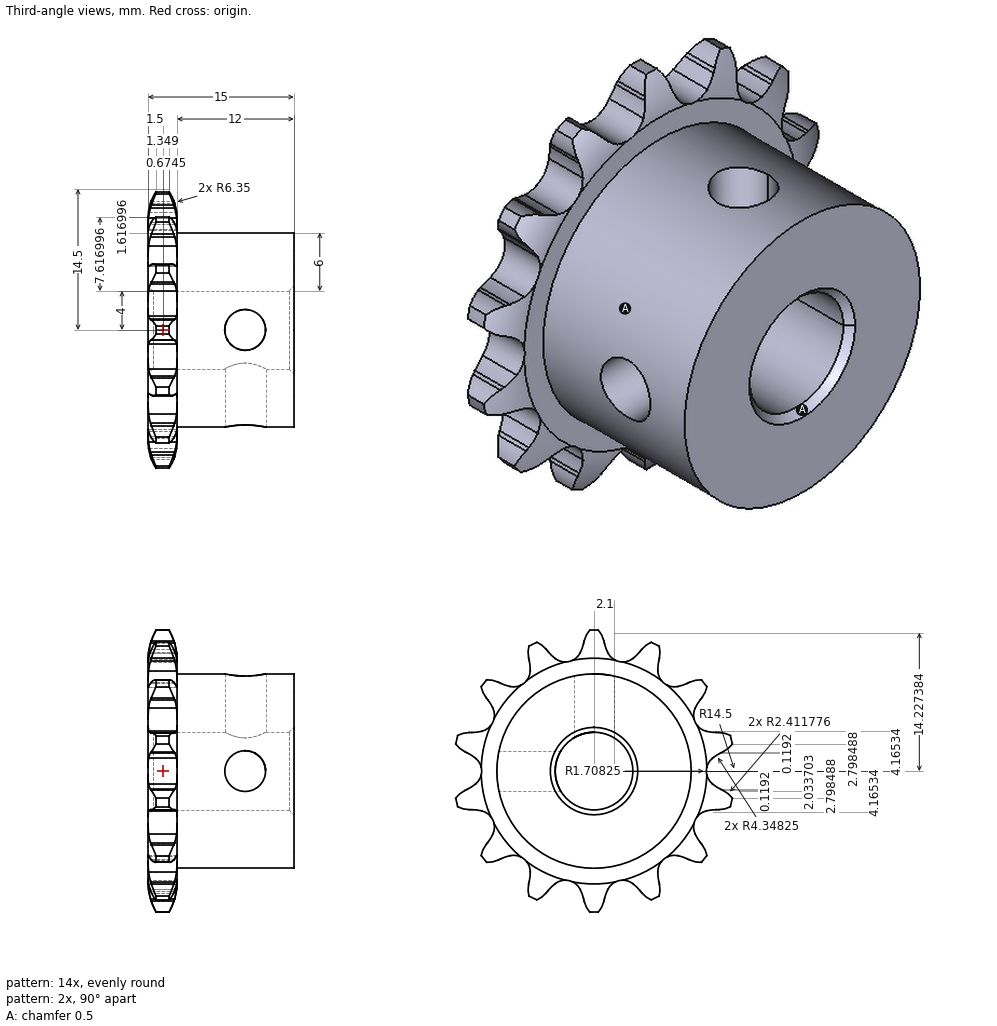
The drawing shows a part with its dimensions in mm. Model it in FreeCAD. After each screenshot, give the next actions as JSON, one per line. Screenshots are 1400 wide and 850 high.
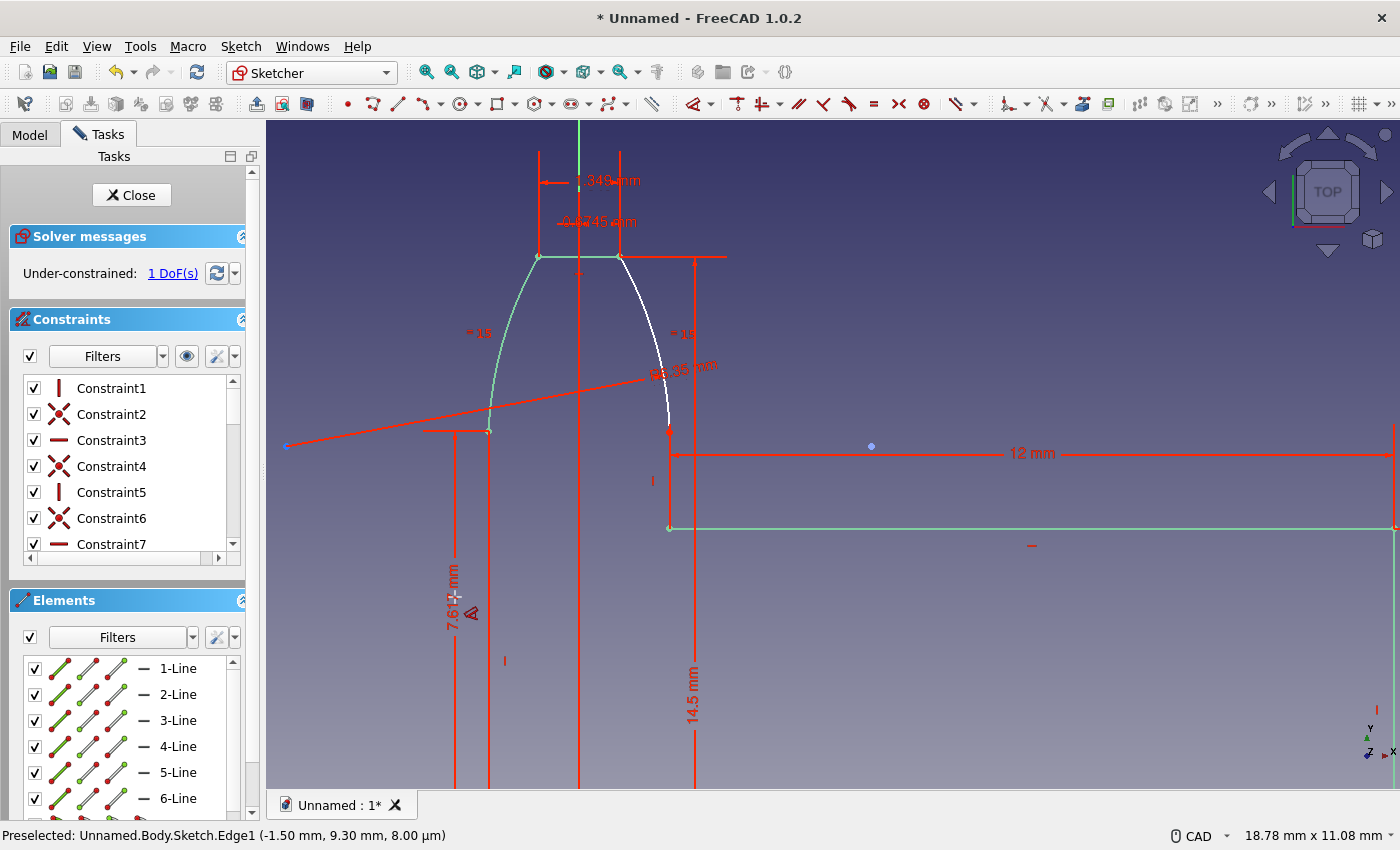
{"action": "left_click", "coordinate": [670, 500]}
{"action": "left_click", "coordinate": [636, 481]}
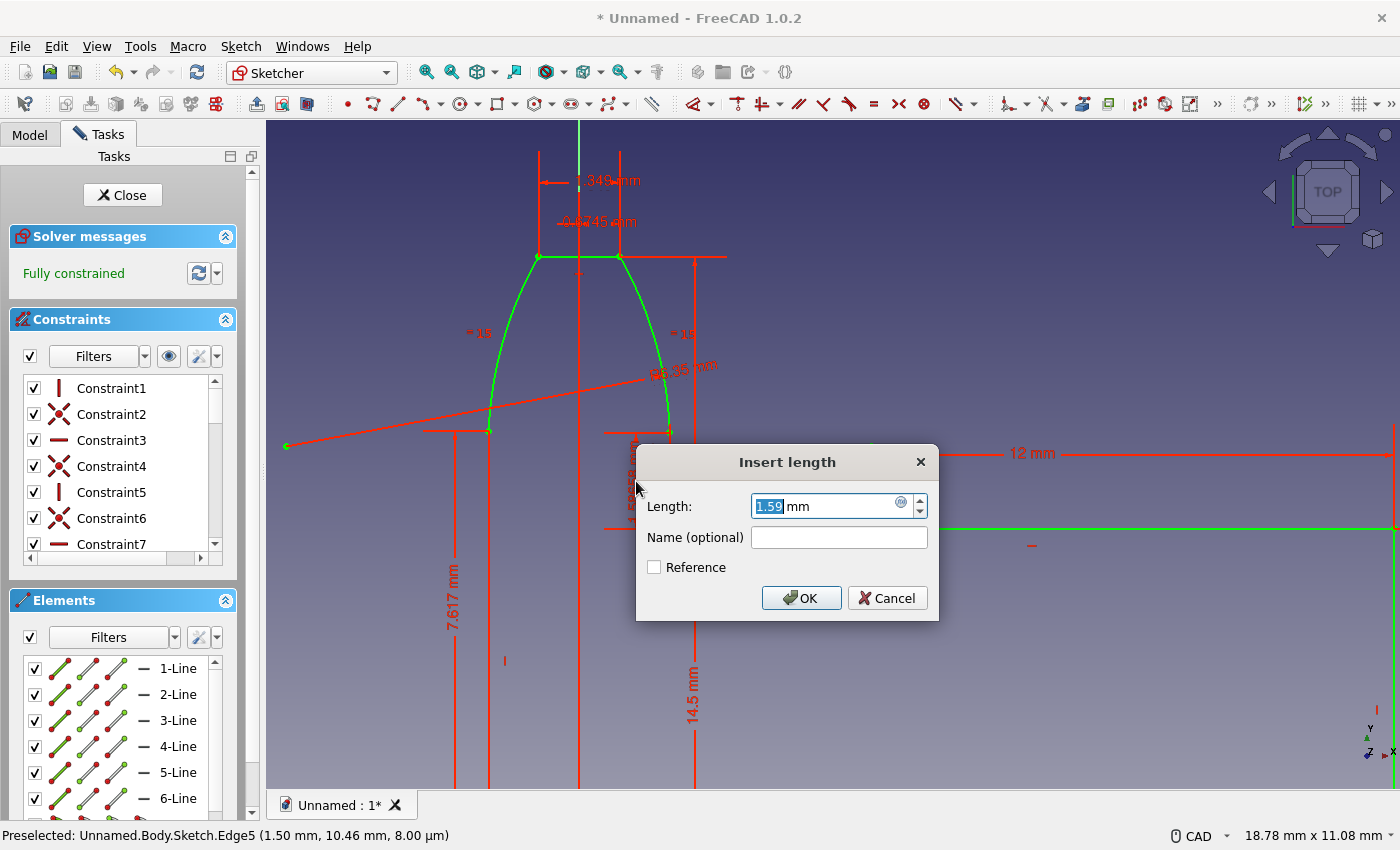
{"action": "type", "text": "1.616996"}
{"action": "key", "text": "Return"}
{"action": "key", "text": "Escape"}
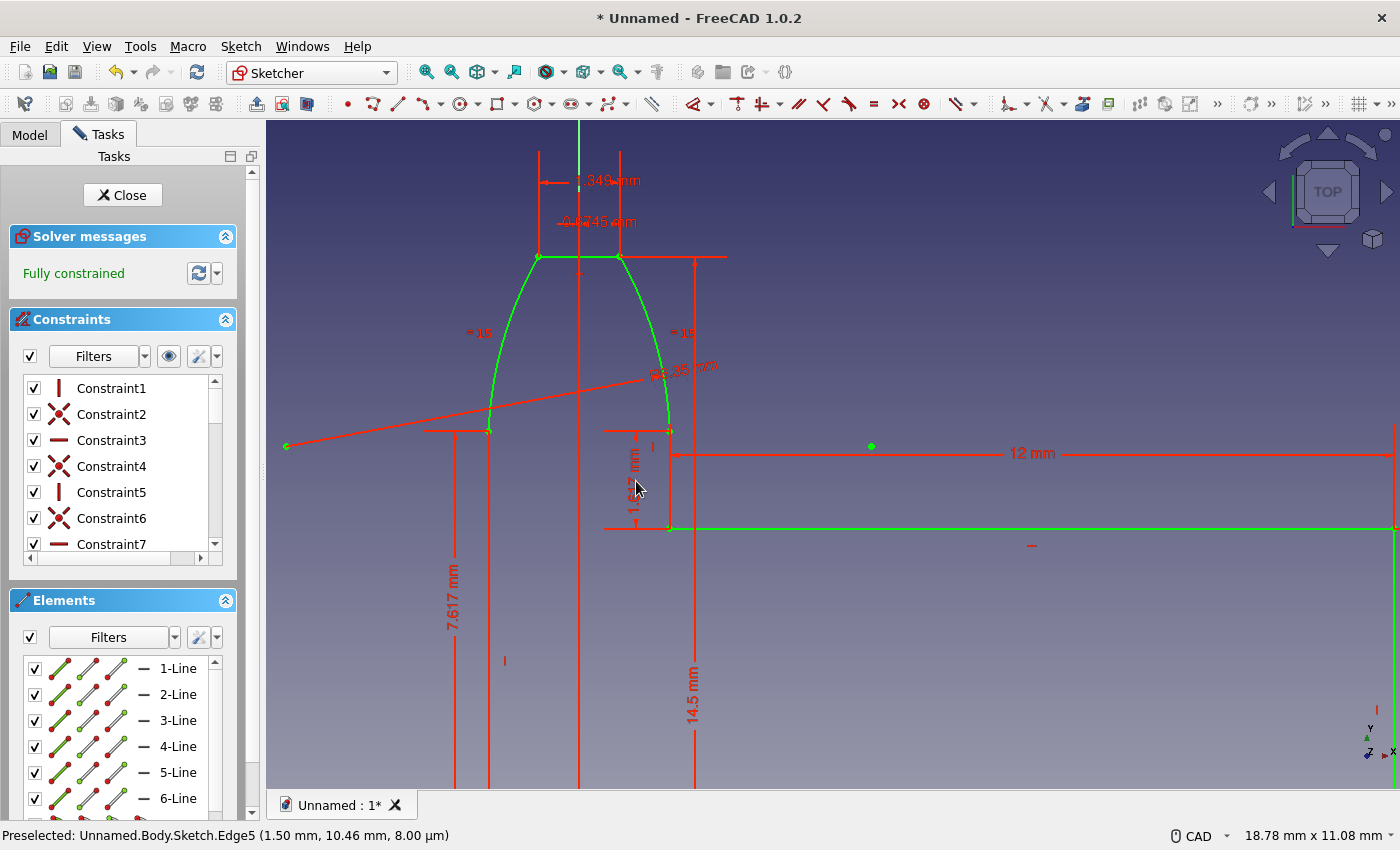
{"action": "left_click", "coordinate": [123, 195]}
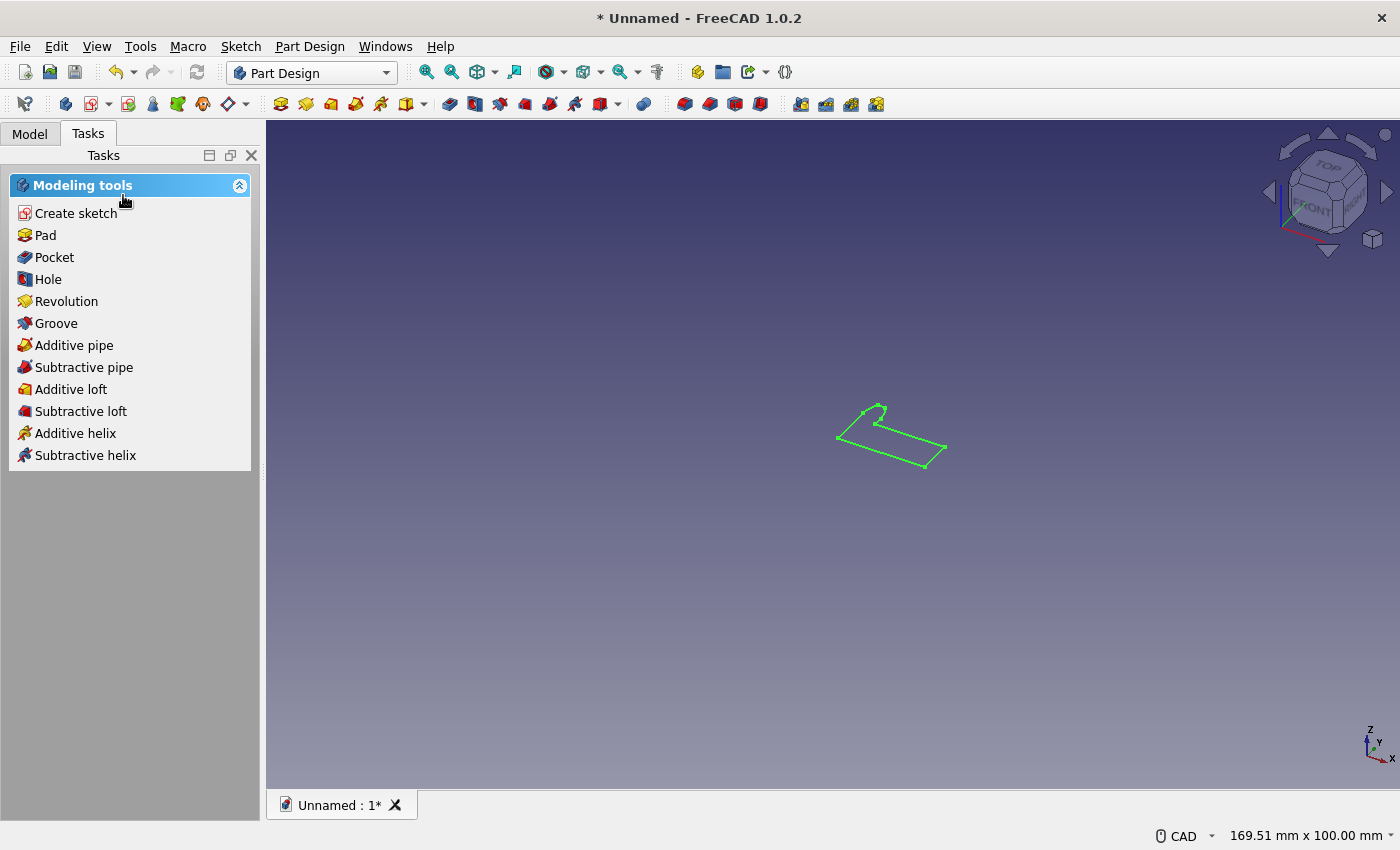
{"action": "left_click", "coordinate": [306, 104]}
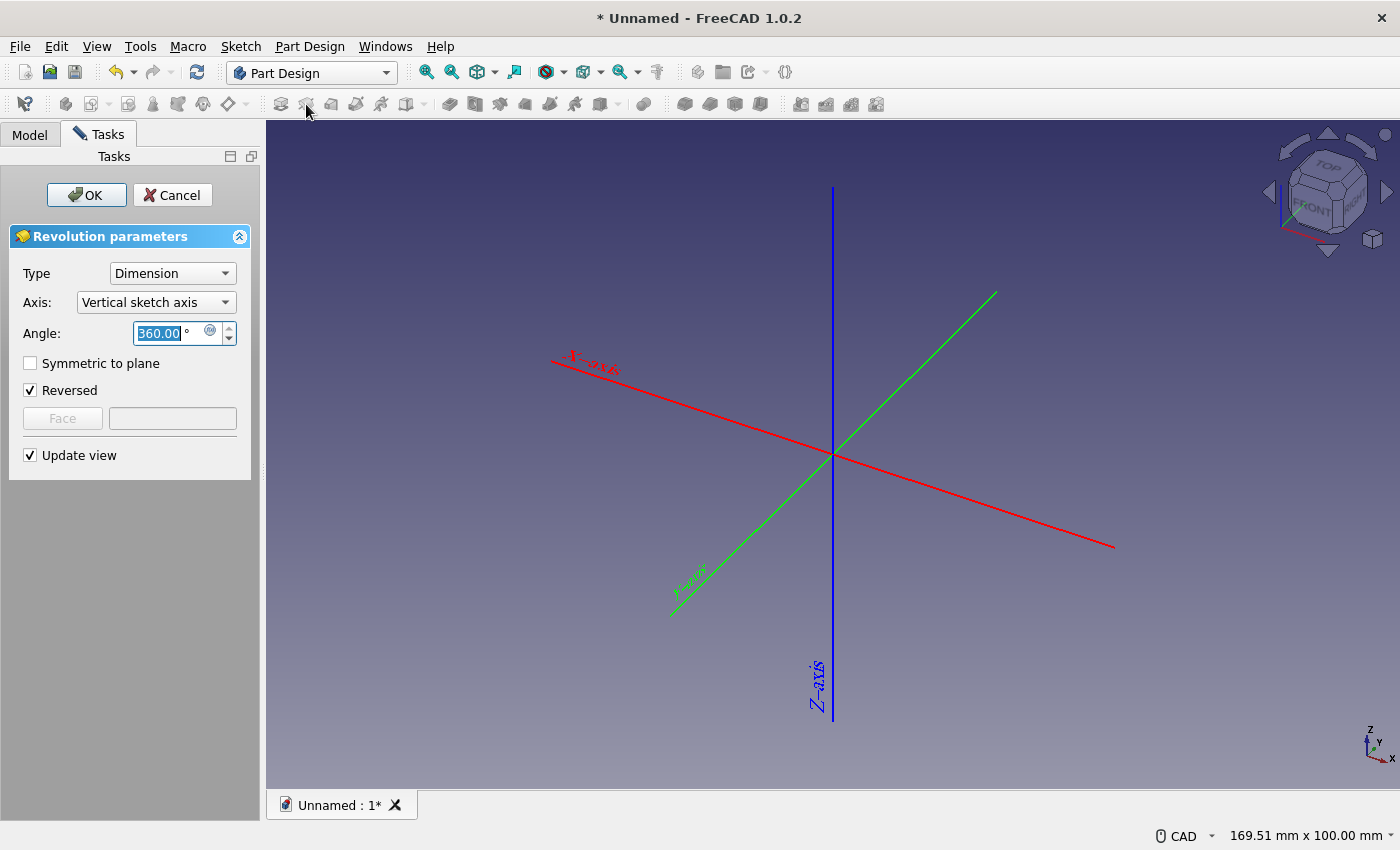
{"action": "left_click", "coordinate": [157, 302]}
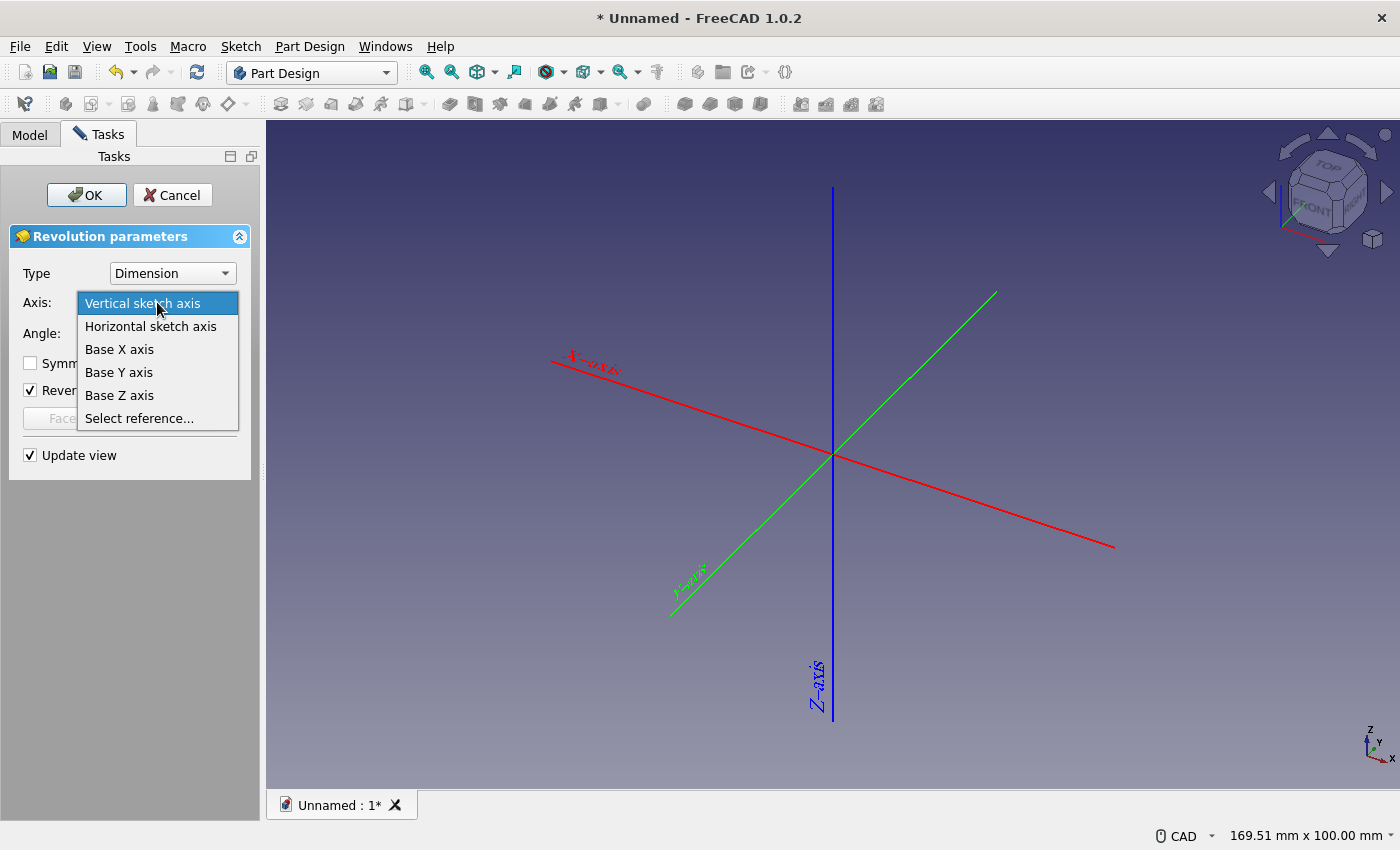
{"action": "left_click", "coordinate": [156, 326]}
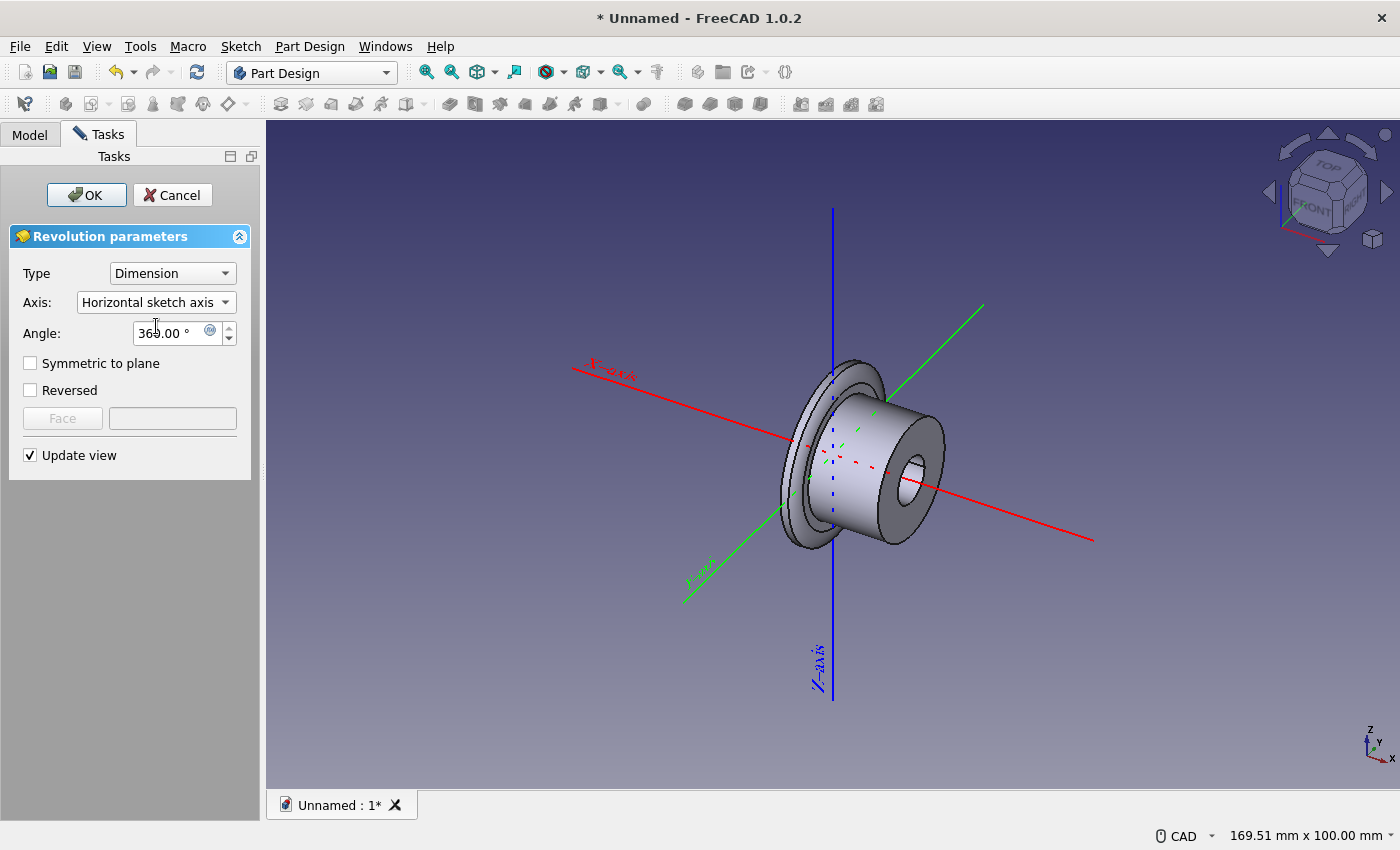
{"action": "left_click", "coordinate": [87, 195]}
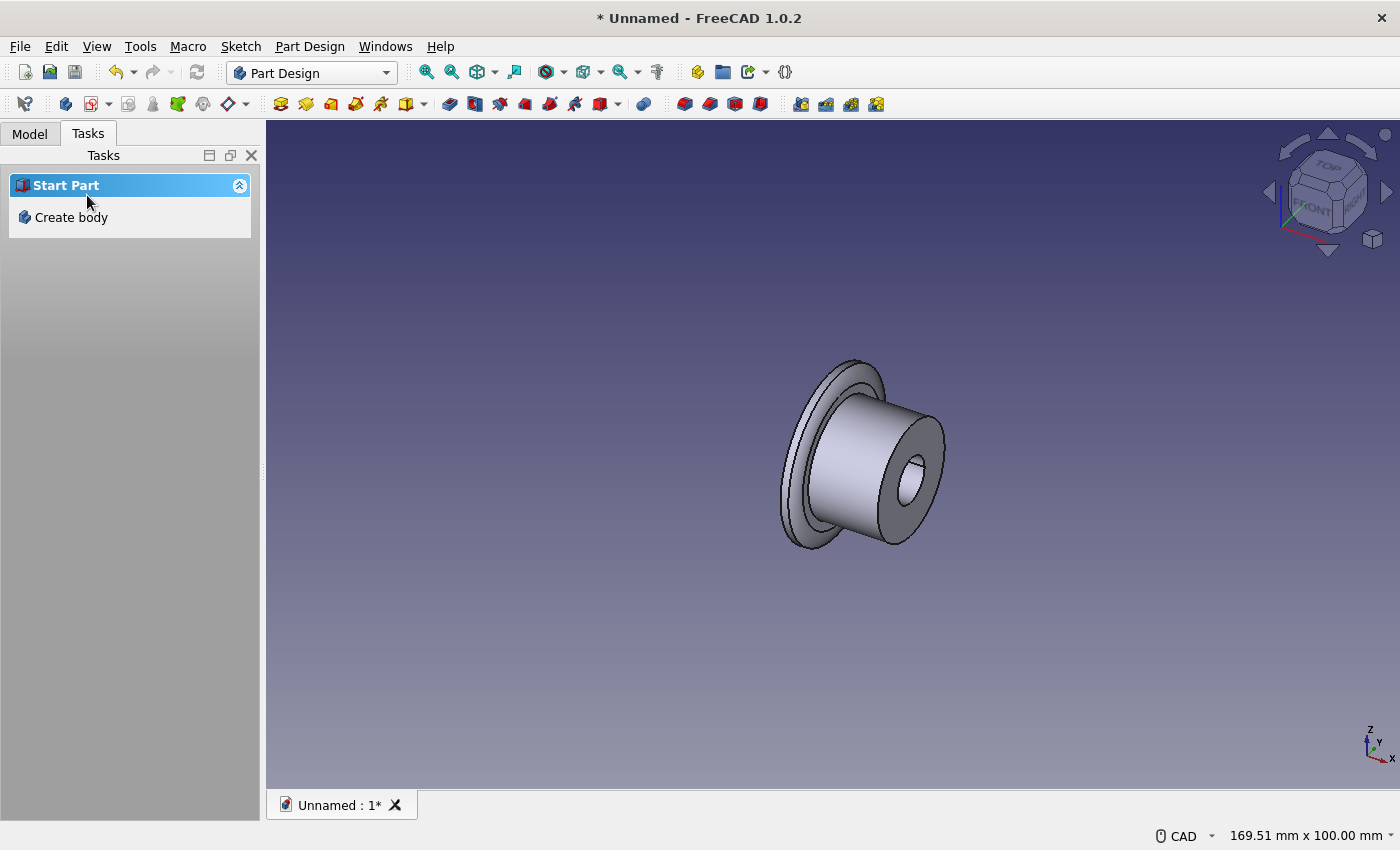
{"action": "left_click", "coordinate": [427, 72]}